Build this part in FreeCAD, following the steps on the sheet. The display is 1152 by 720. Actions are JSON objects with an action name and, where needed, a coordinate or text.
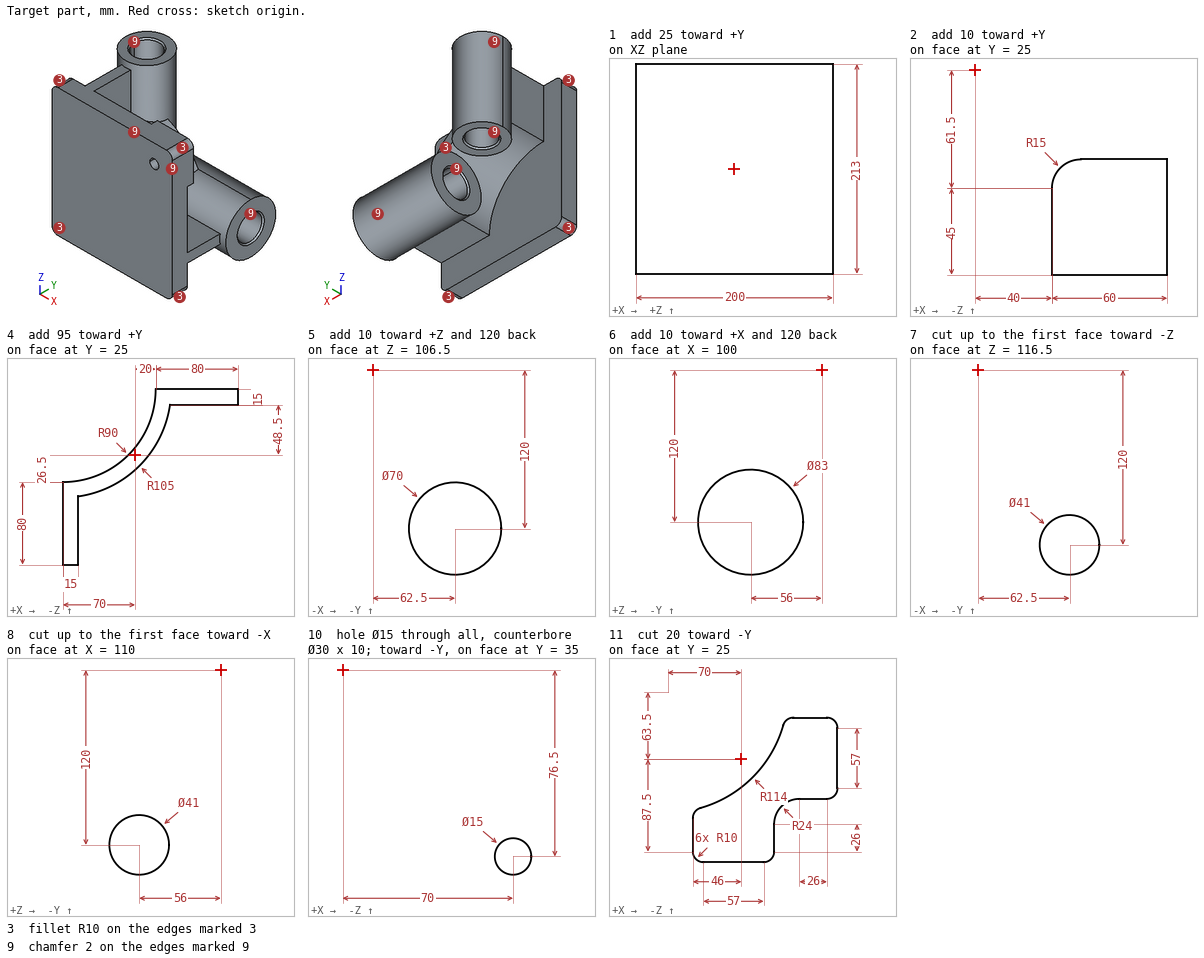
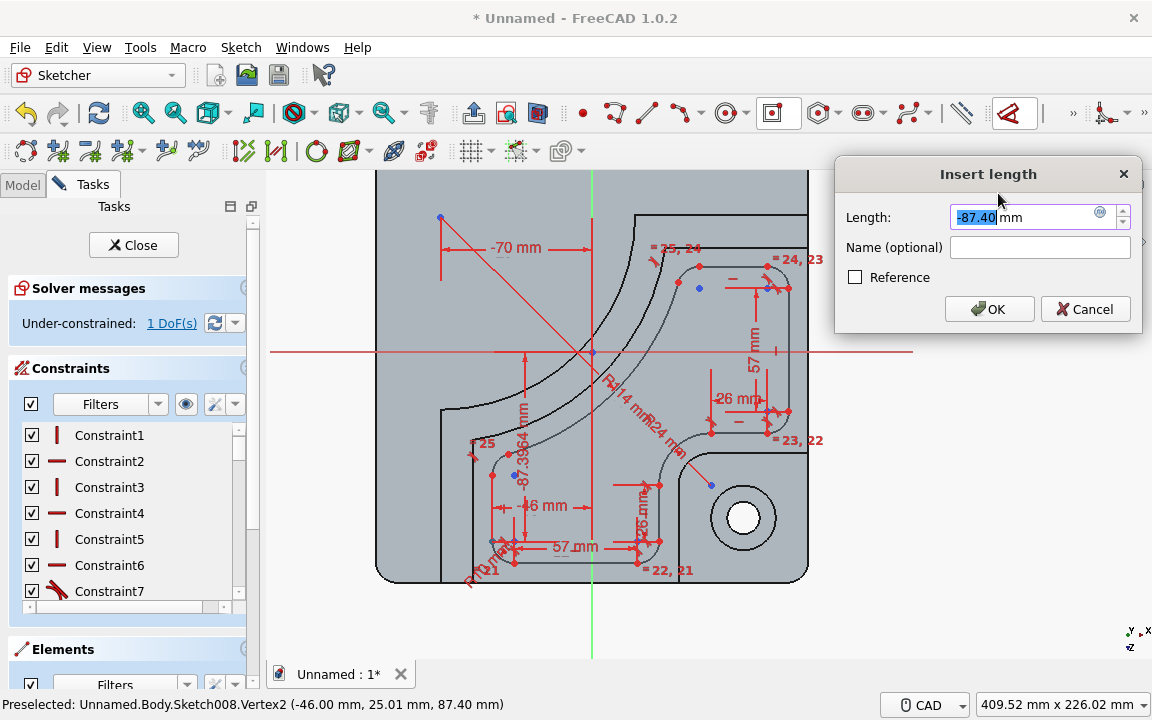
{"action": "type", "text": "-87.5"}
{"action": "key", "text": "Return"}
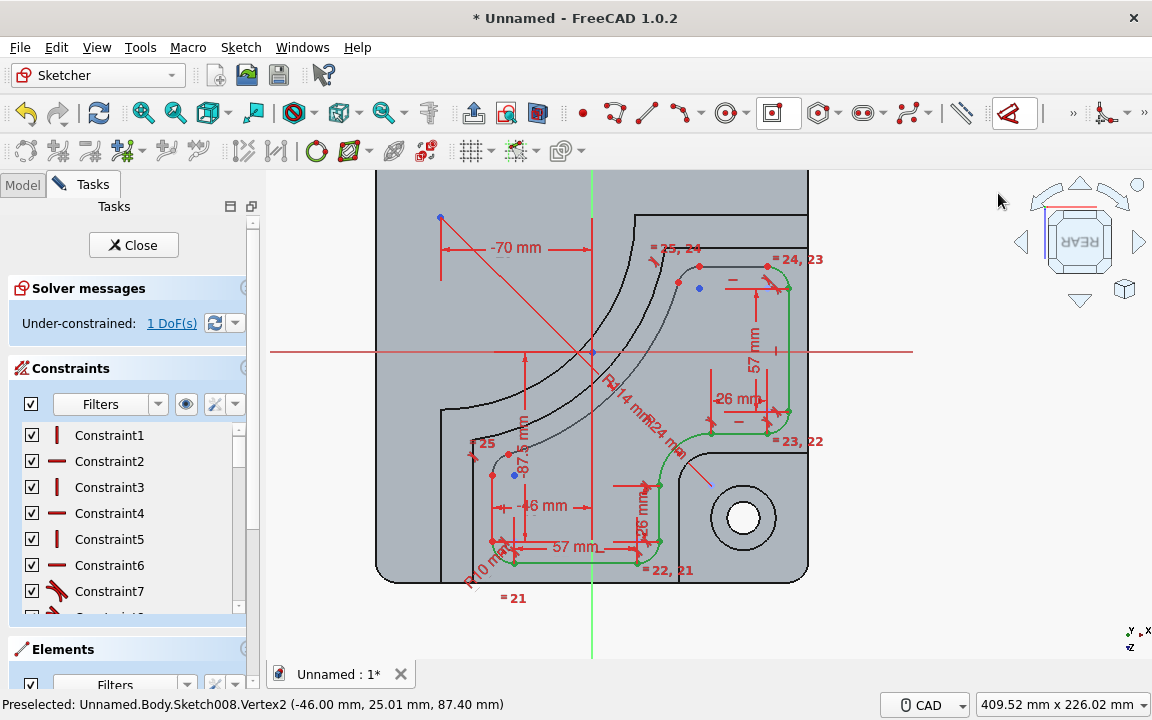
{"action": "left_click", "coordinate": [441, 217]}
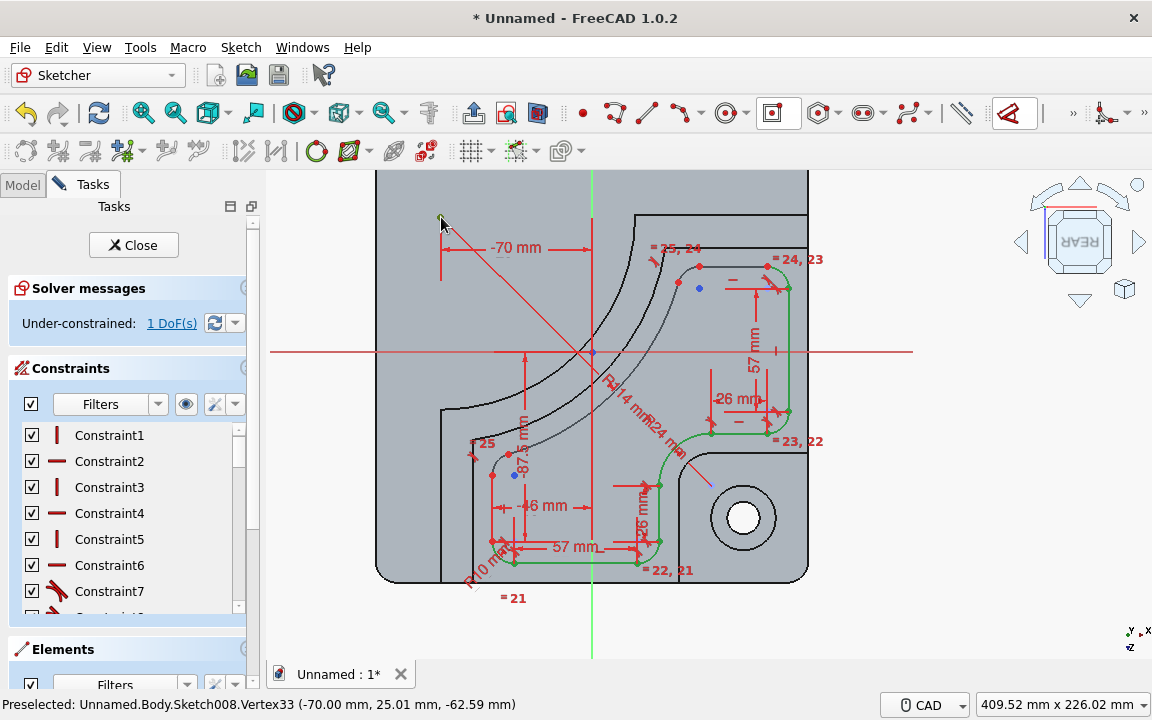
{"action": "left_click", "coordinate": [1032, 114]}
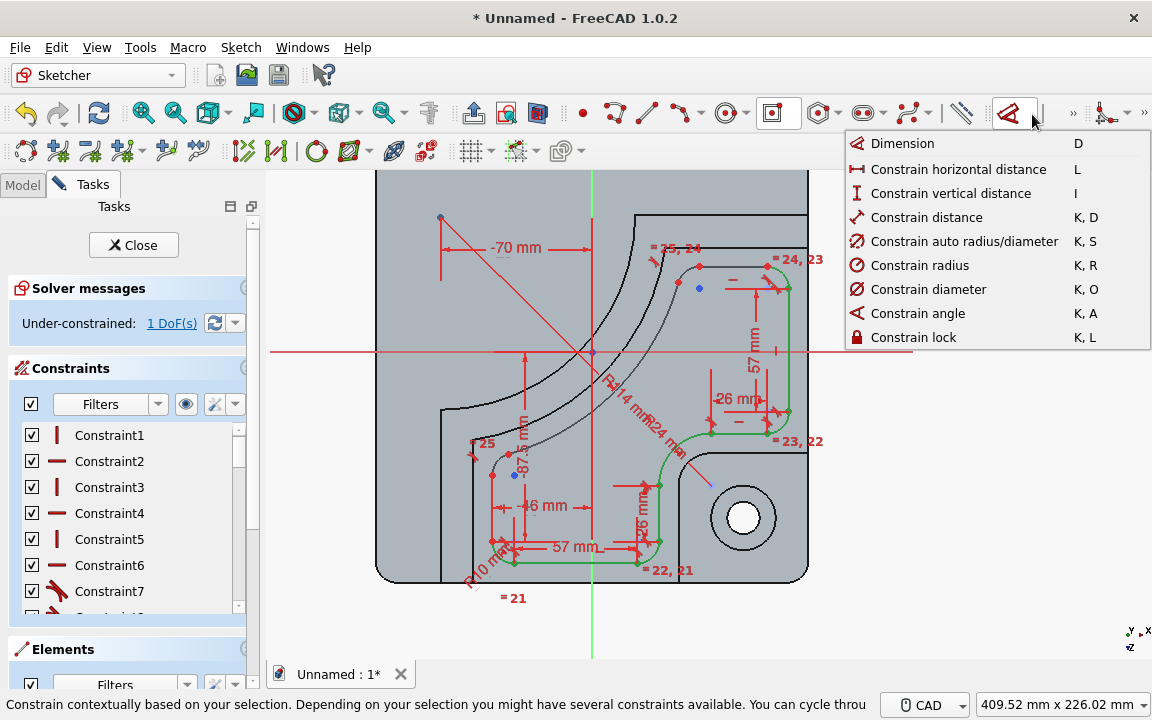
{"action": "left_click", "coordinate": [998, 193]}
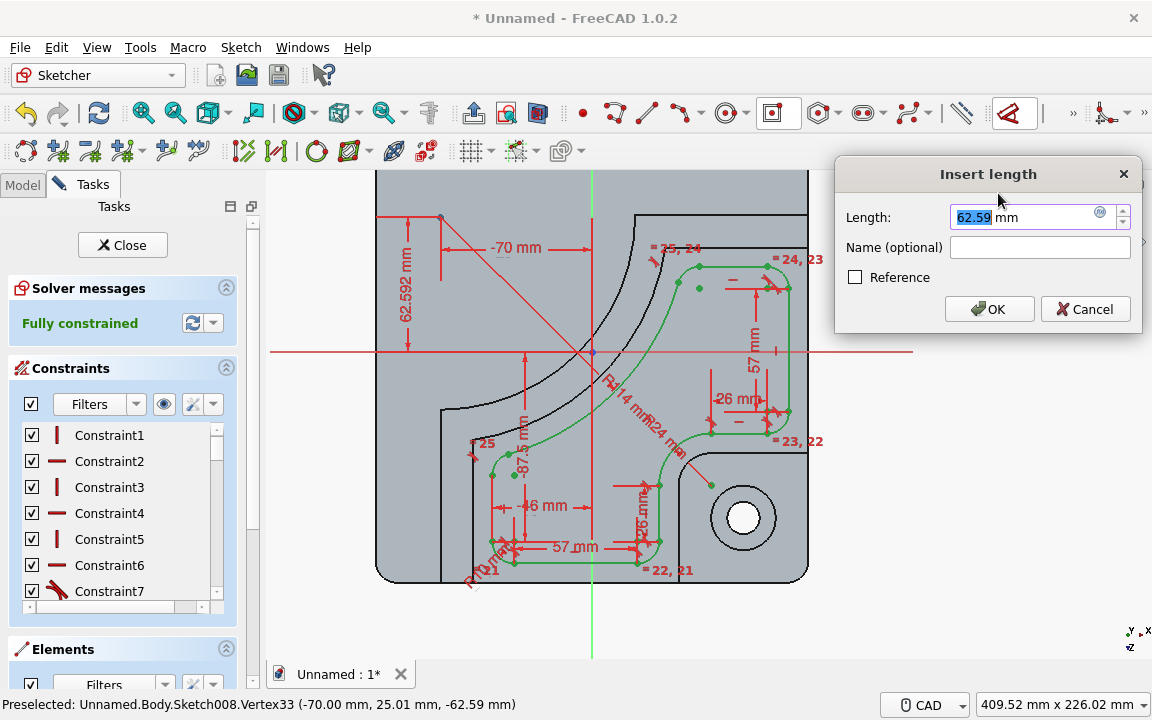
{"action": "type", "text": "63.5"}
{"action": "key", "text": "Return"}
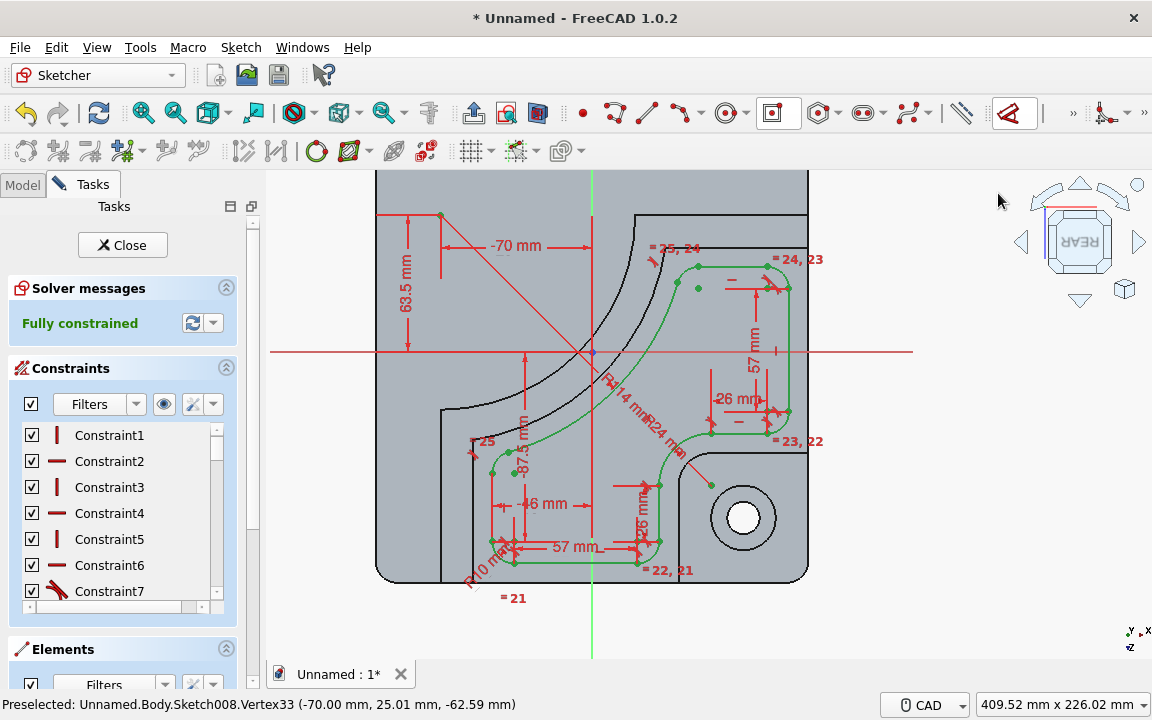
{"action": "left_click", "coordinate": [123, 245]}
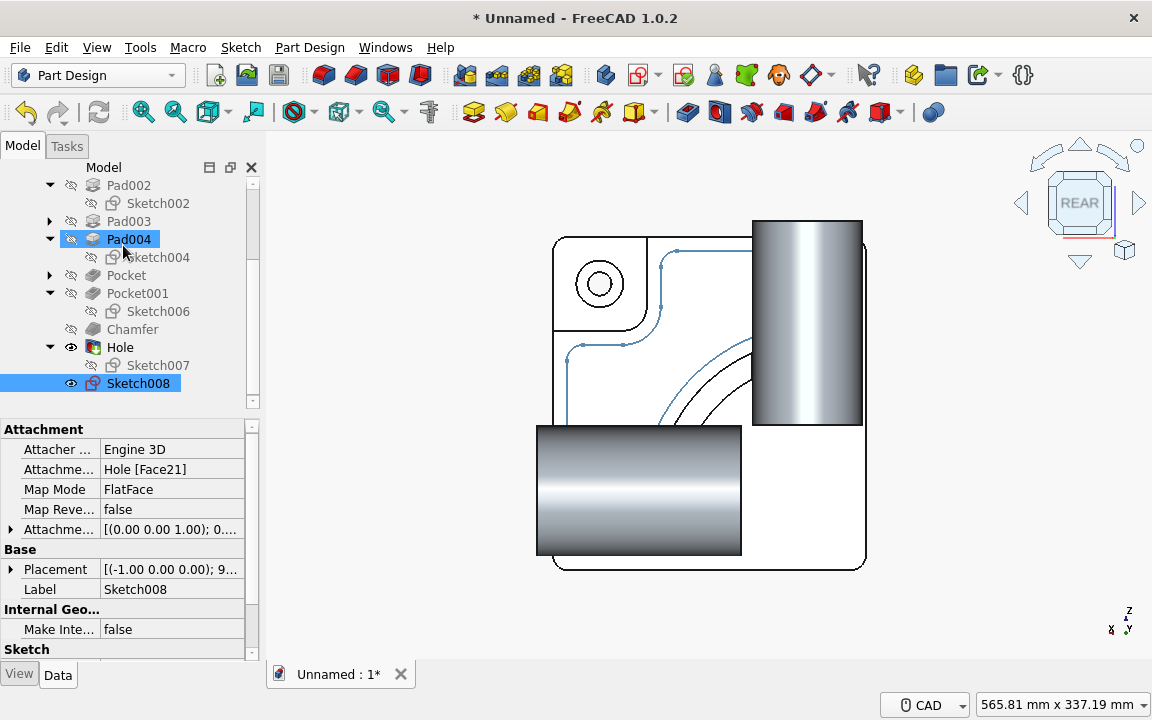
{"action": "left_click", "coordinate": [688, 112]}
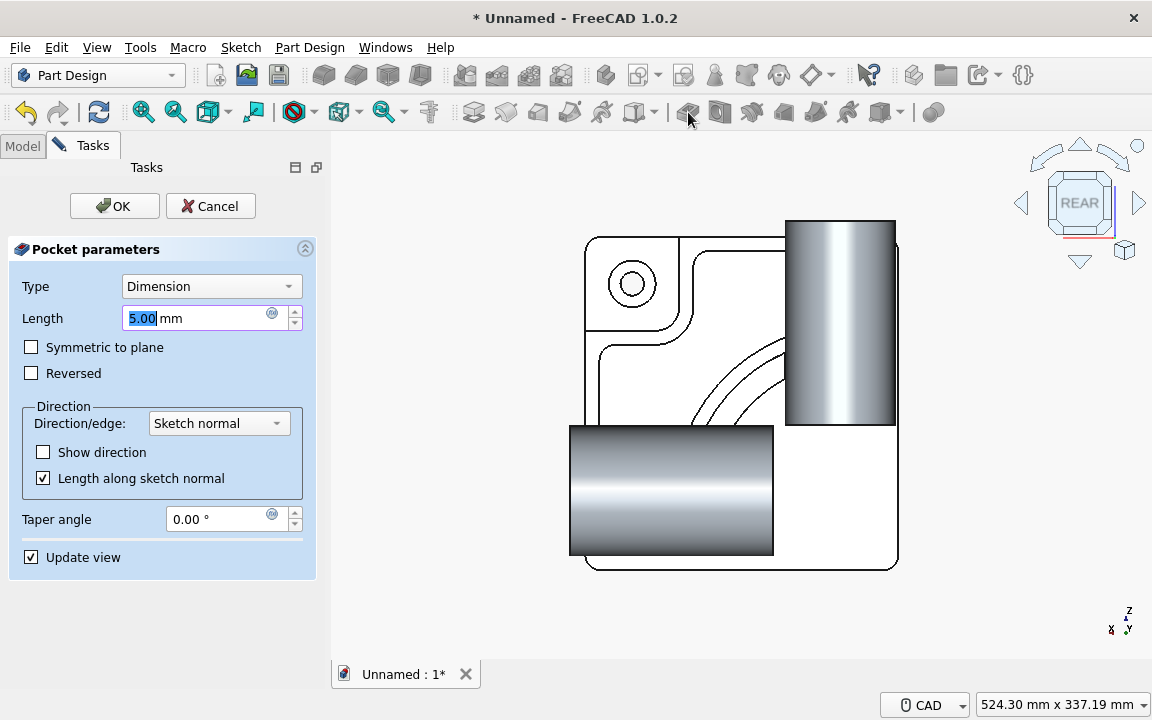
{"action": "type", "text": "20"}
{"action": "key", "text": "Tab"}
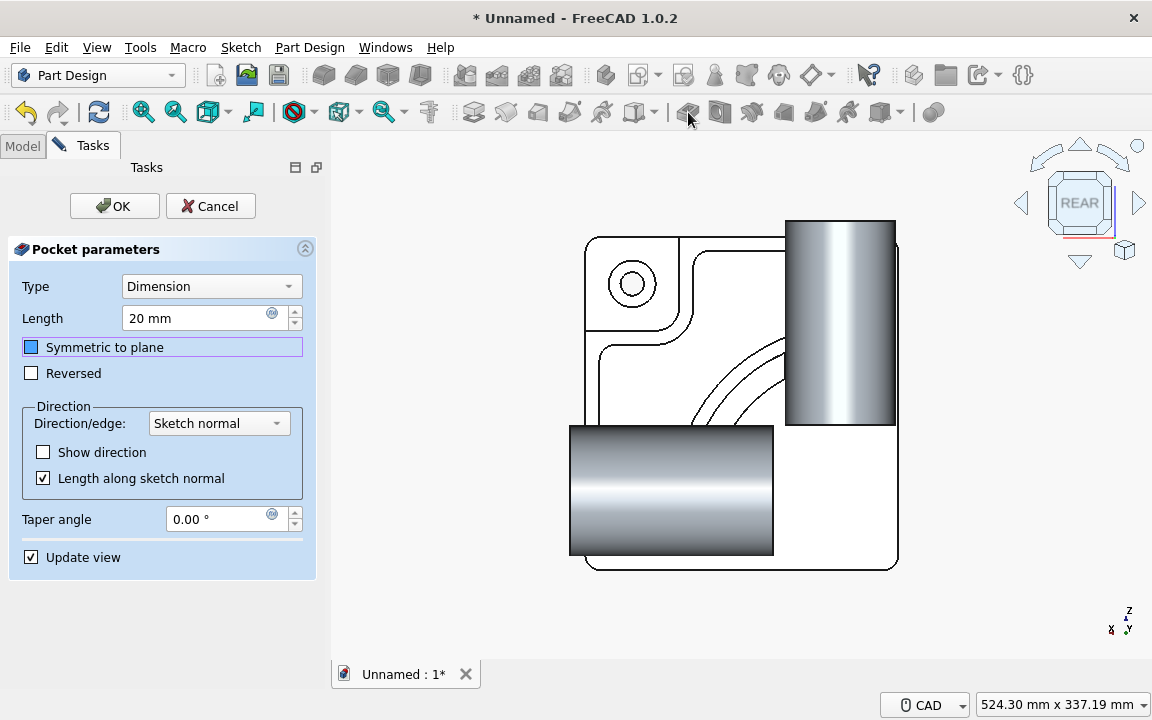
{"action": "left_click", "coordinate": [115, 206]}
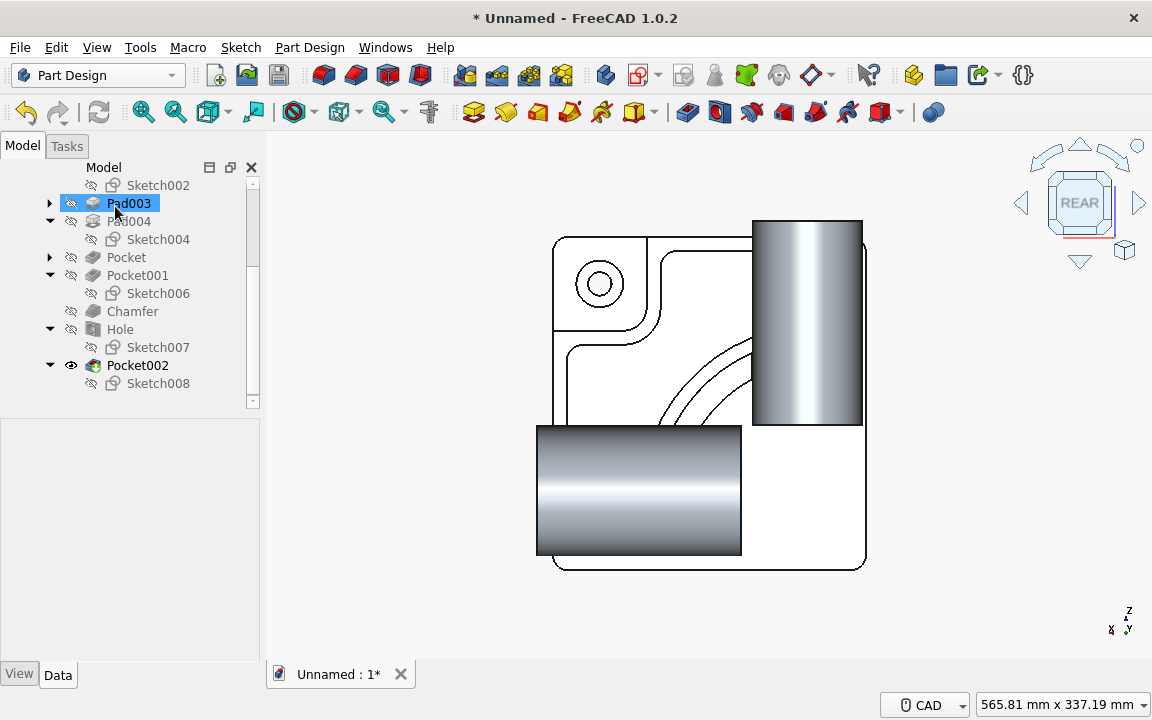
{"action": "key", "text": "0"}